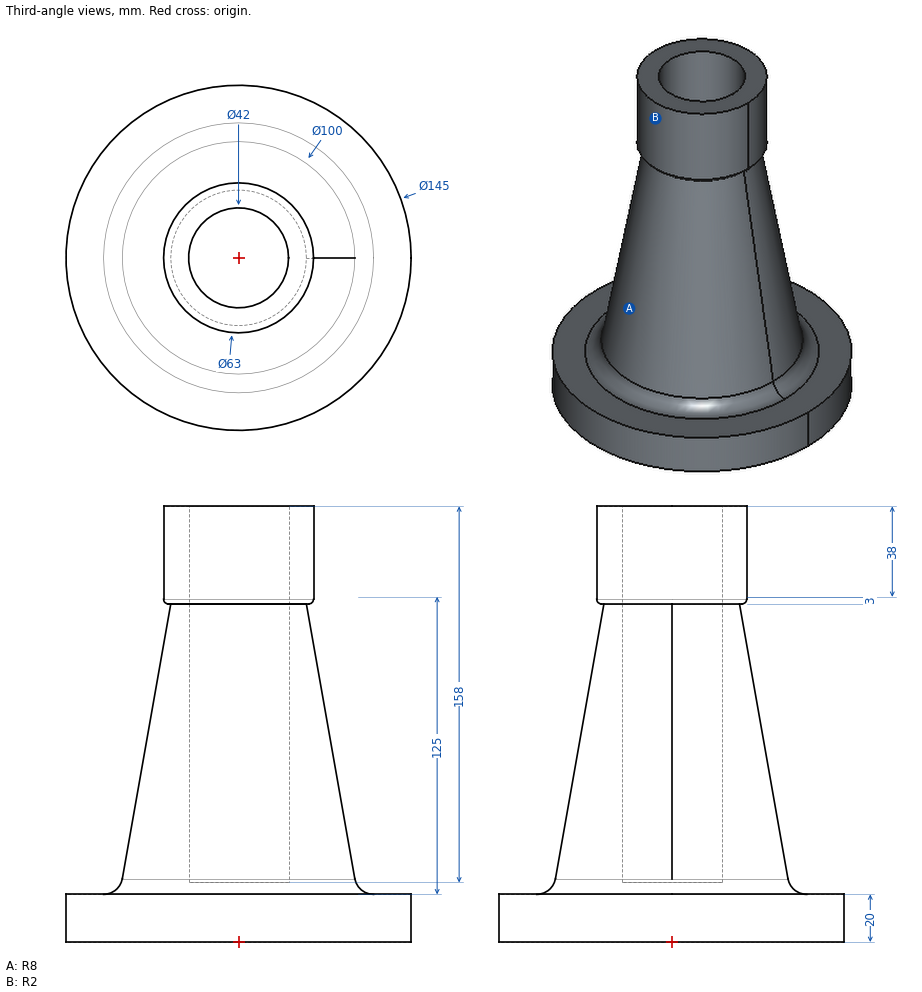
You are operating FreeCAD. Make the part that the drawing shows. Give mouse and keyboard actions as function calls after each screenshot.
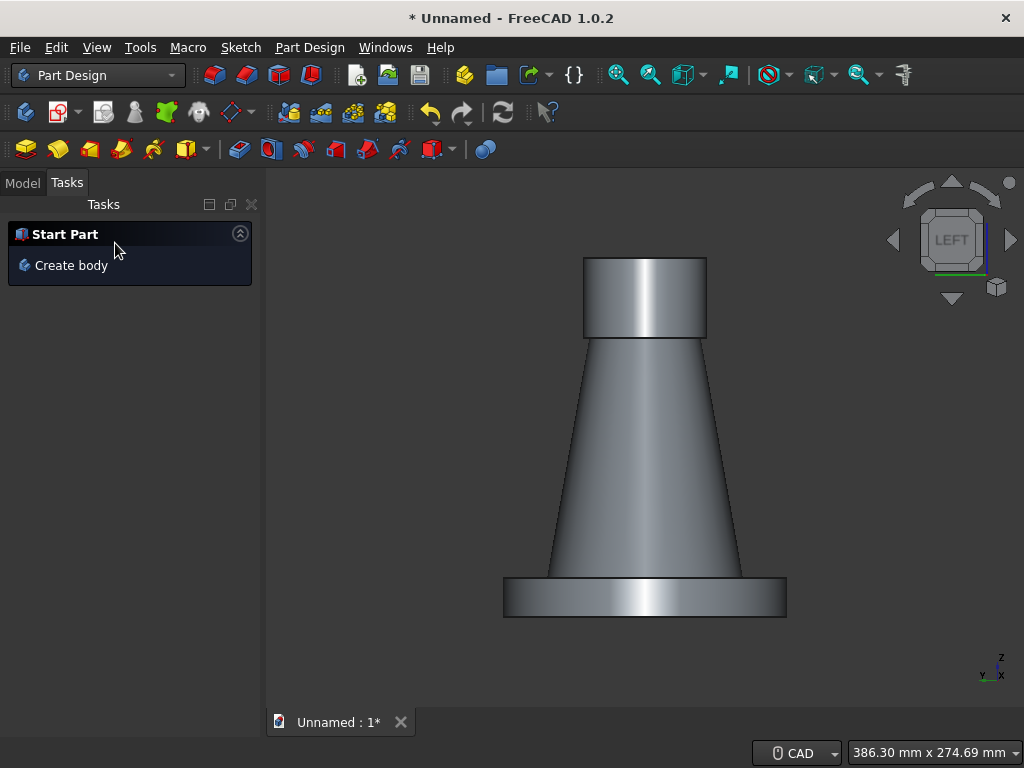
key(v)
key(3)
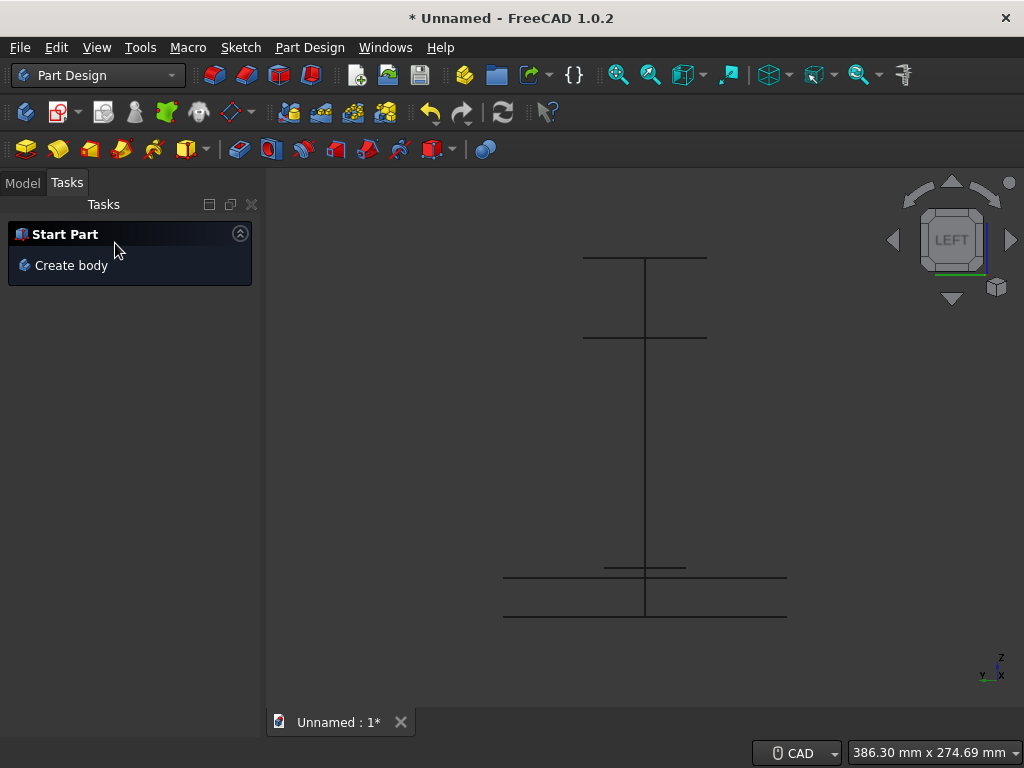
key(0)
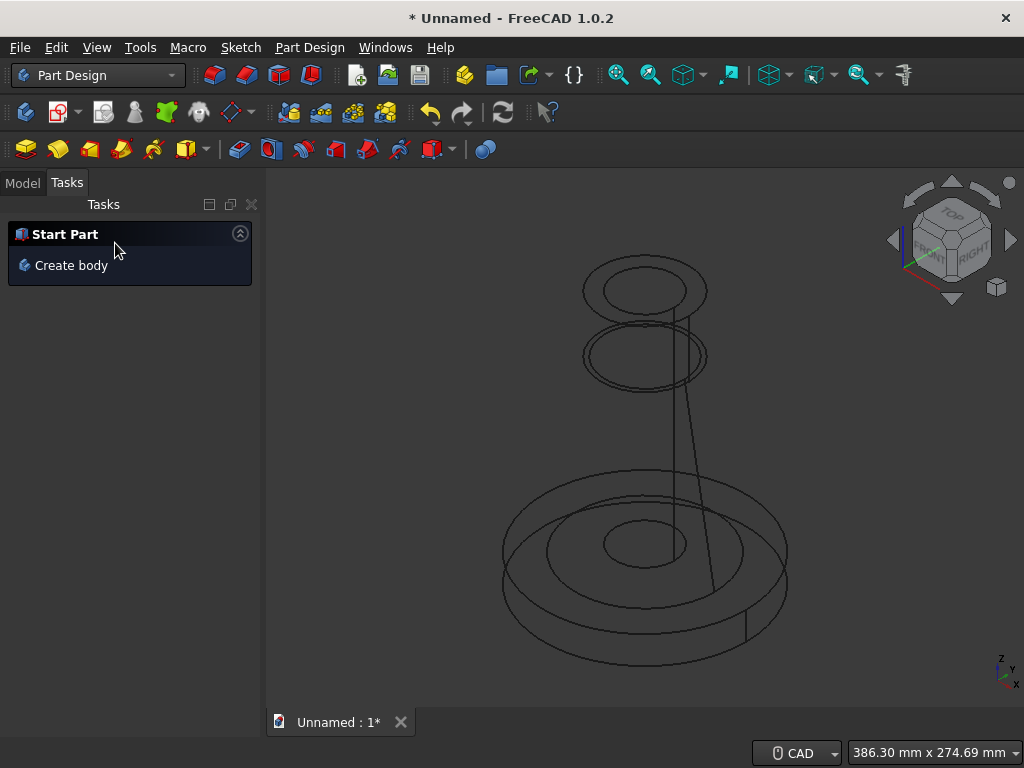
click(576, 511)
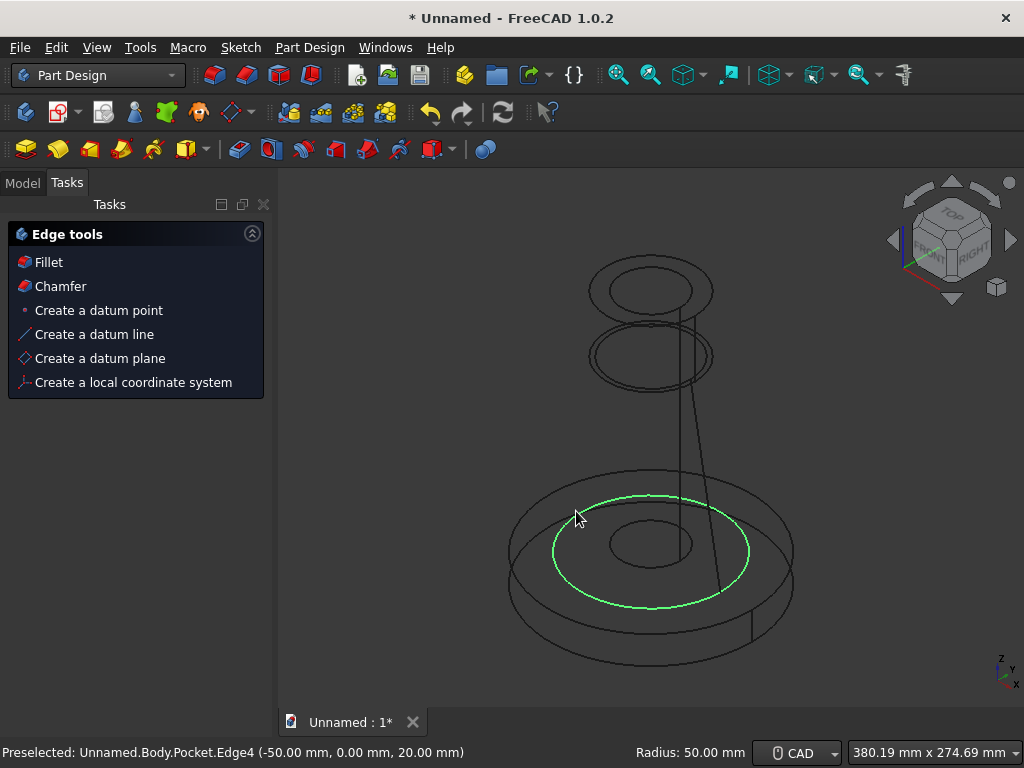
key(v)
key(1)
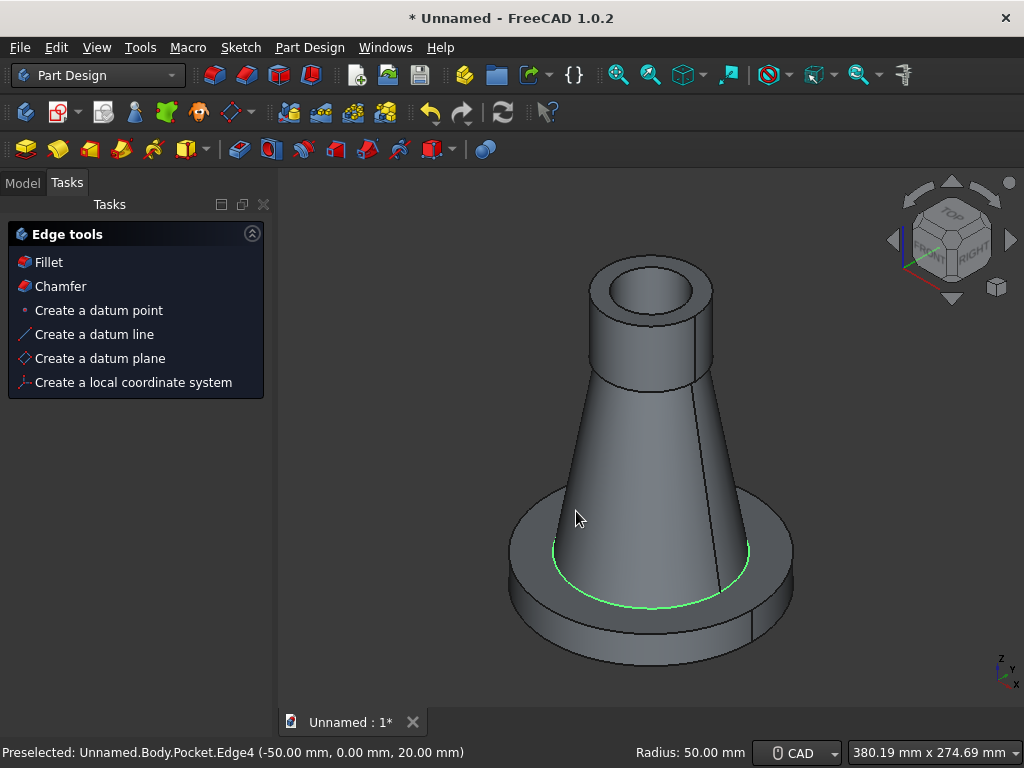
click(216, 76)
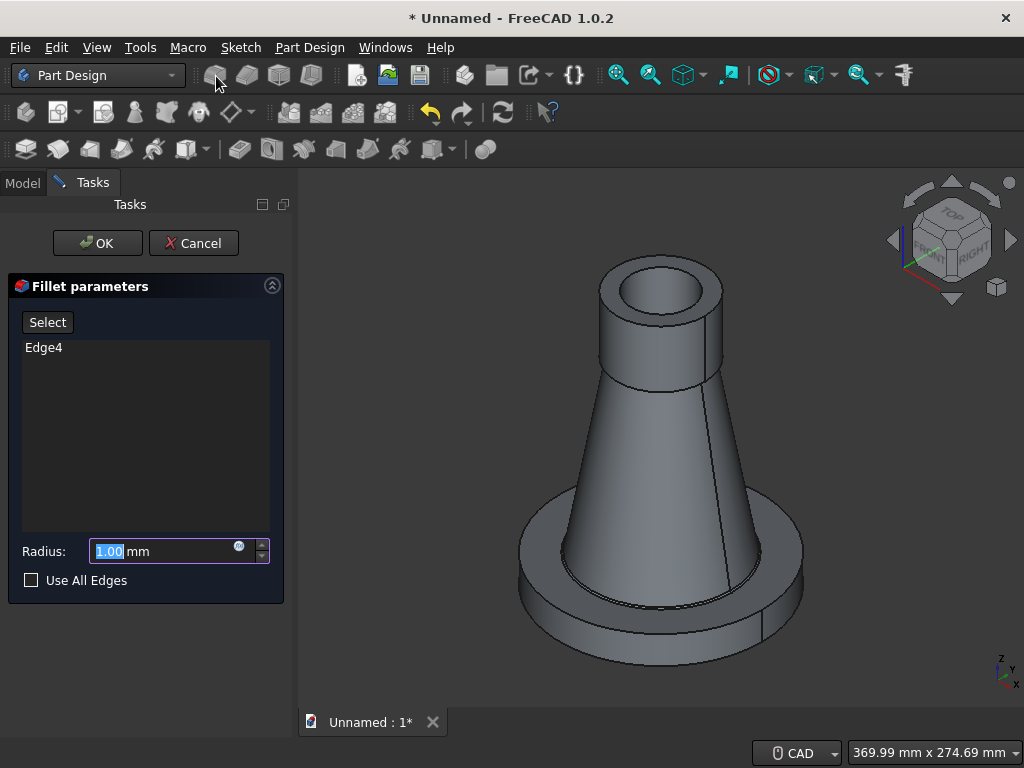
text(8)
key(Tab)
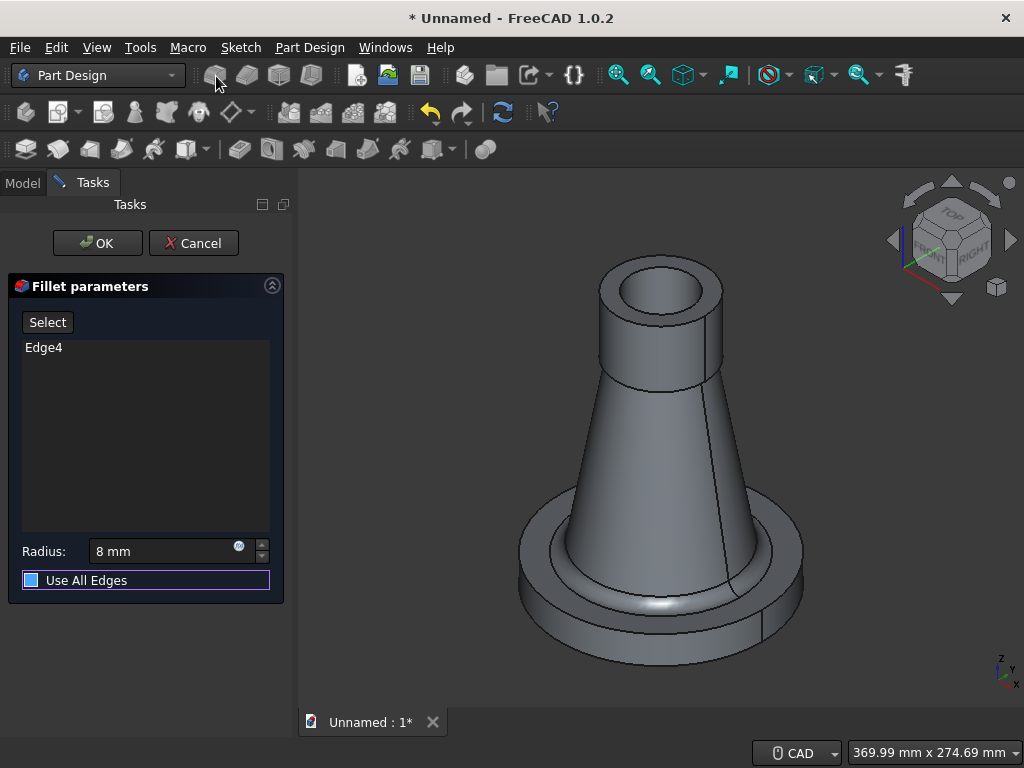
click(98, 243)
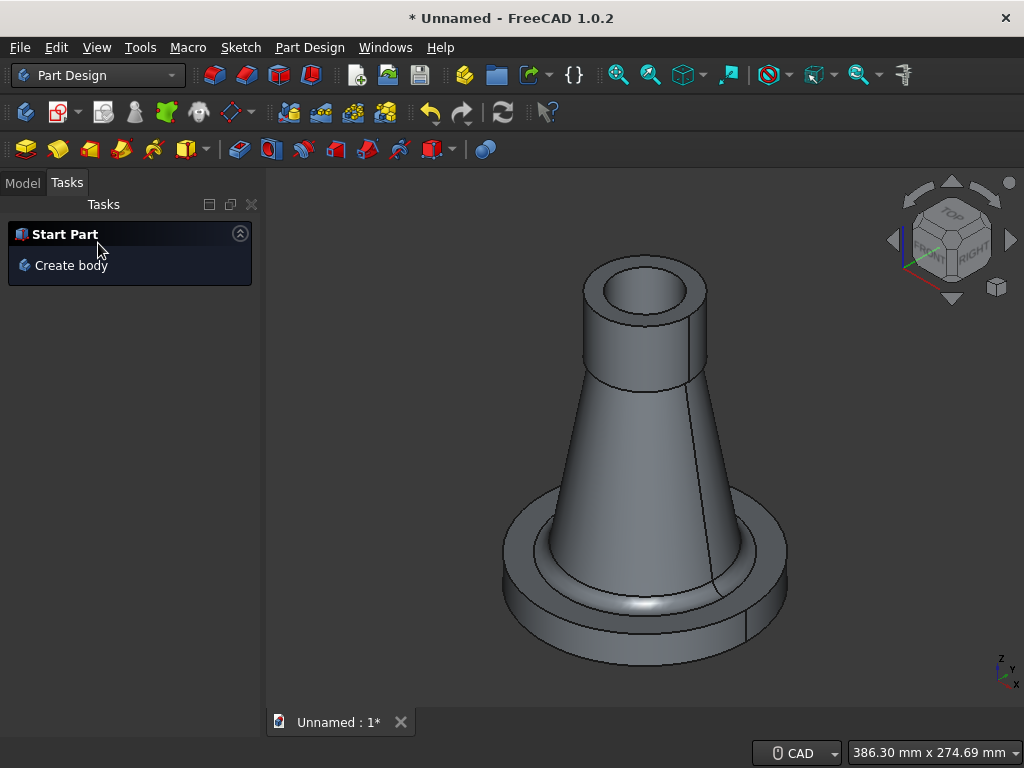
key(2)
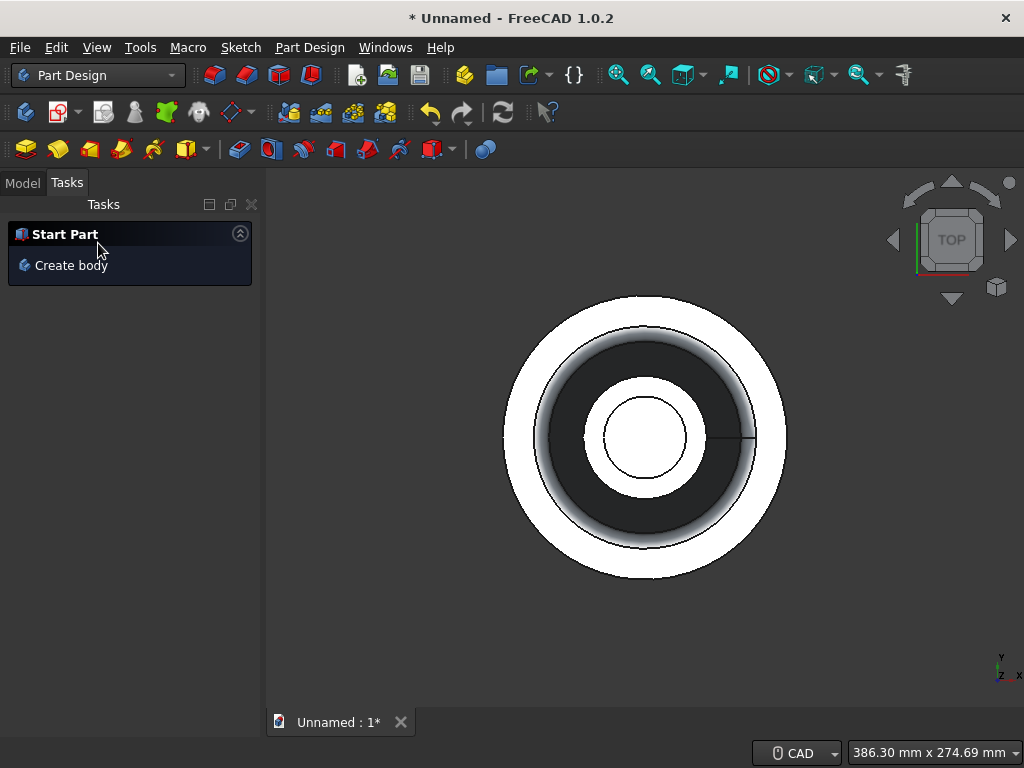
key(0)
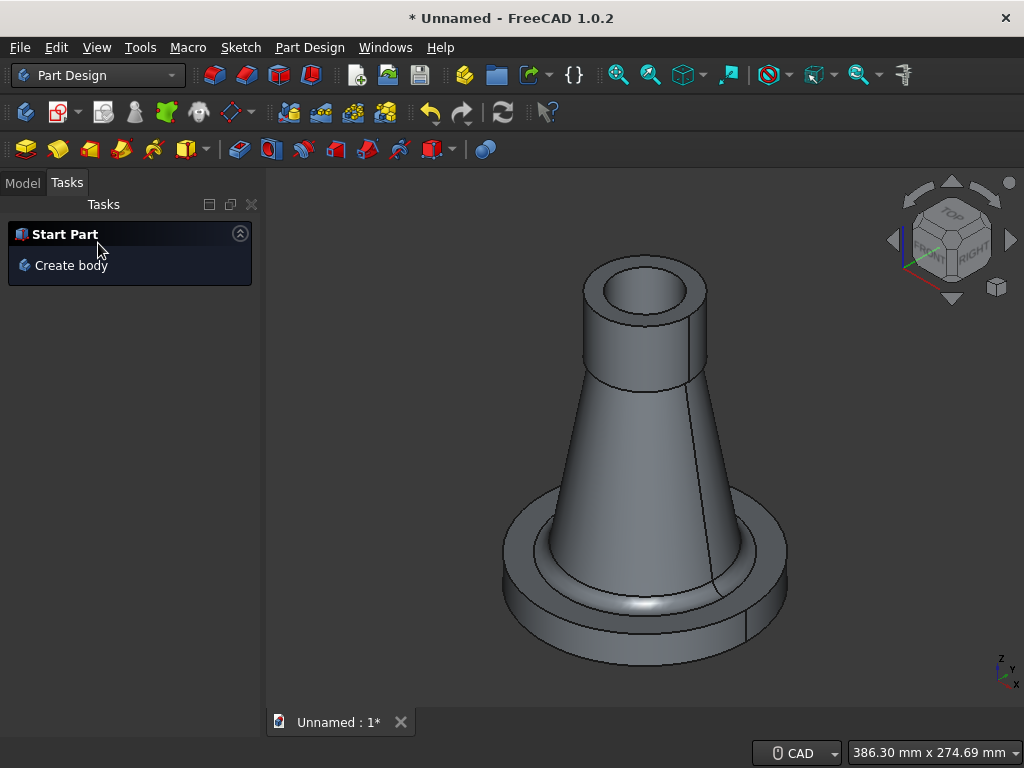
key(1)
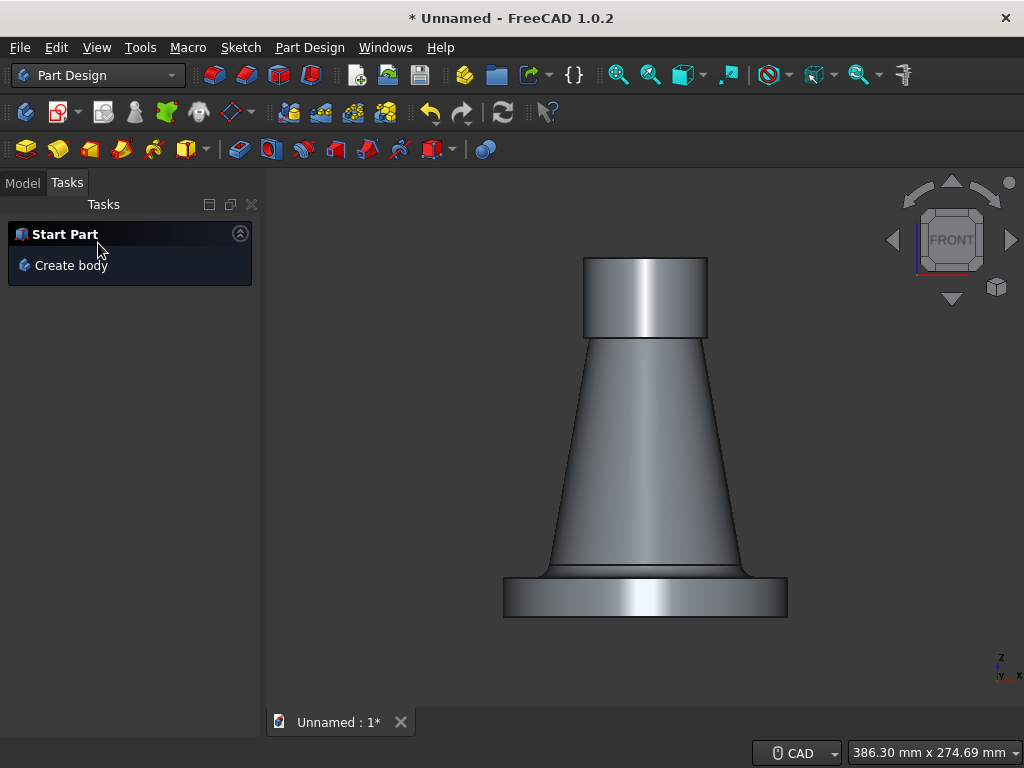
click(595, 337)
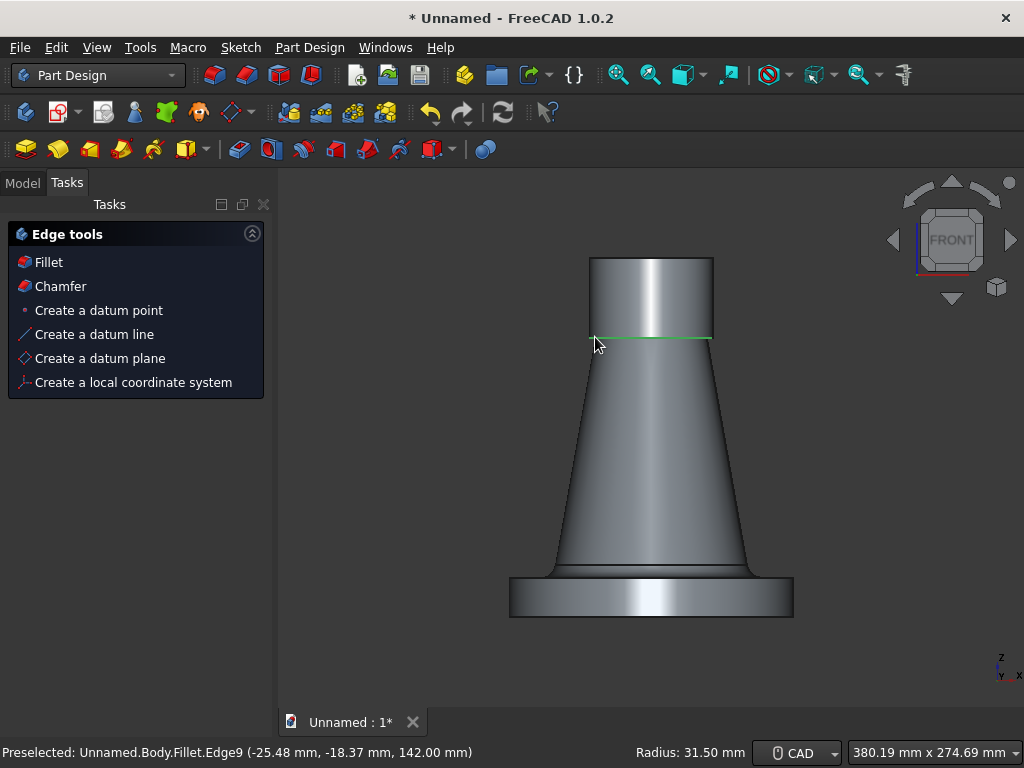
click(216, 76)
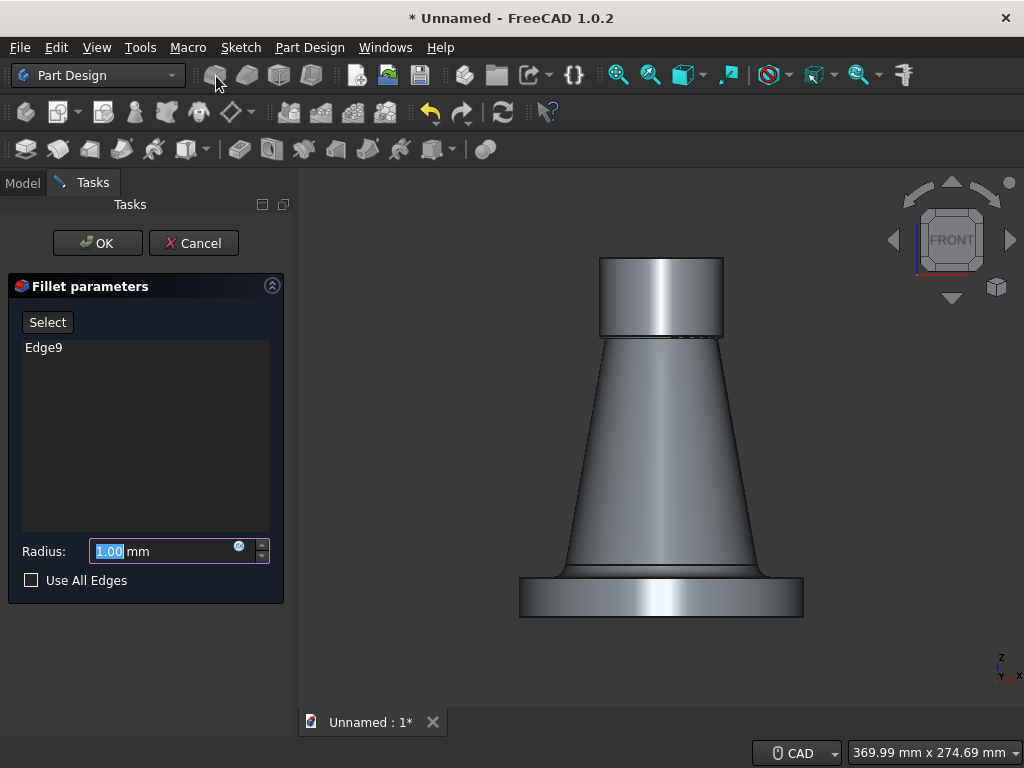
text(2)
key(Tab)